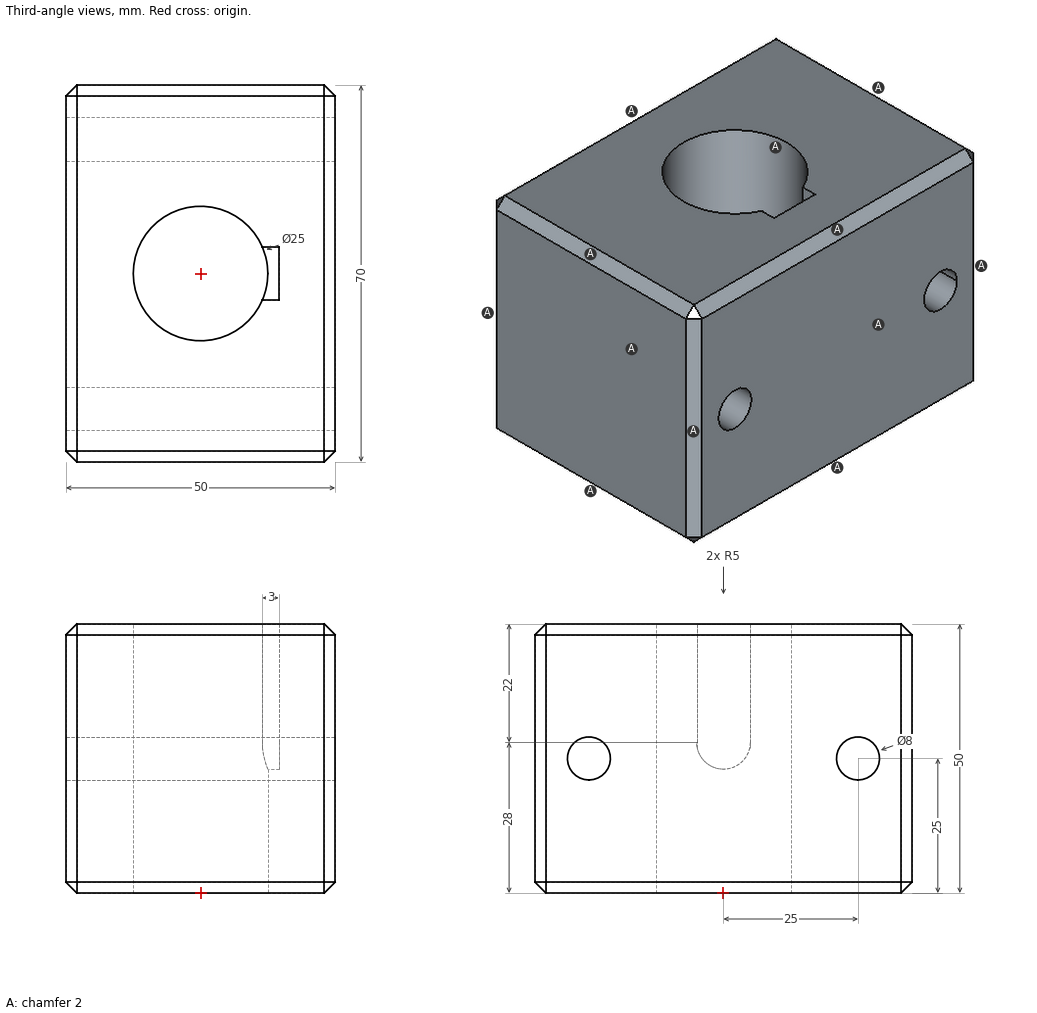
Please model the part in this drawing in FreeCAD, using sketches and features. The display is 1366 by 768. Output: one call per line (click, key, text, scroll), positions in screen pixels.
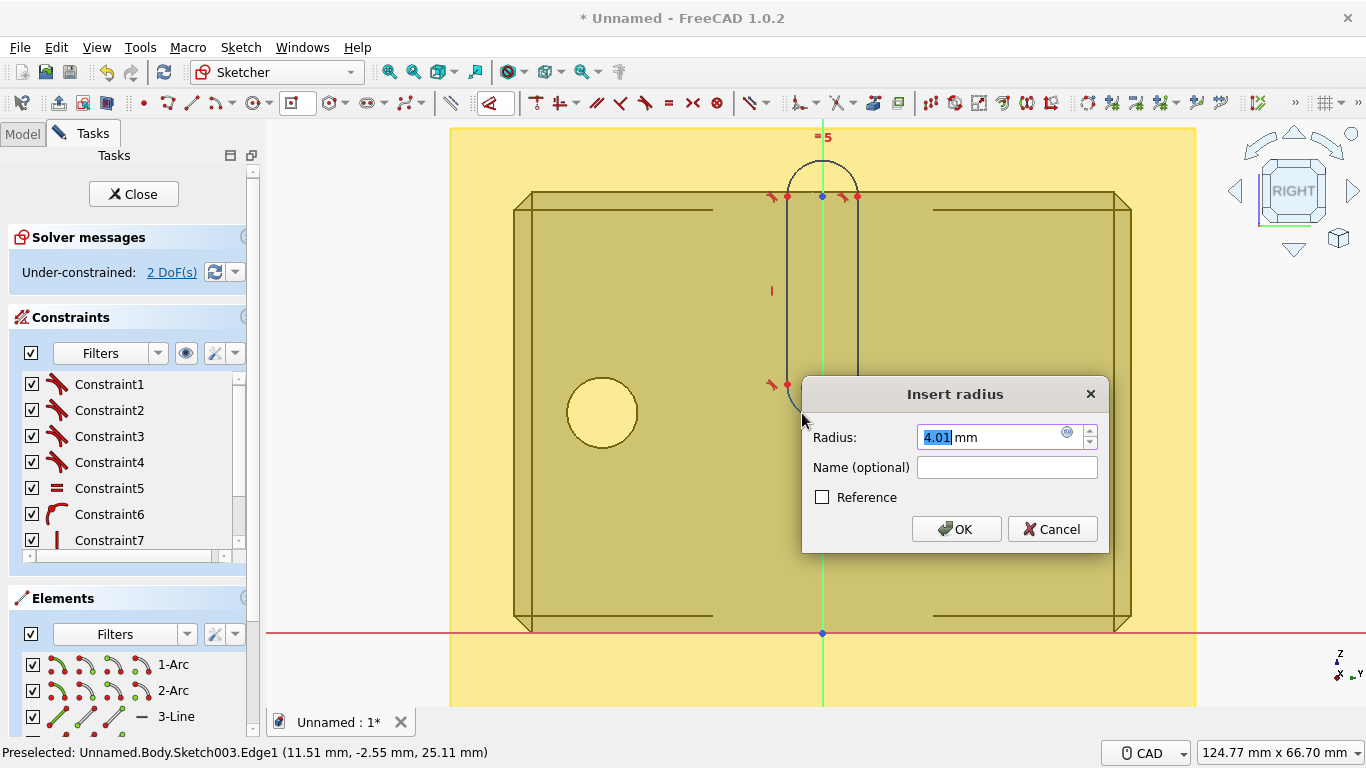
text(5)
key(Return)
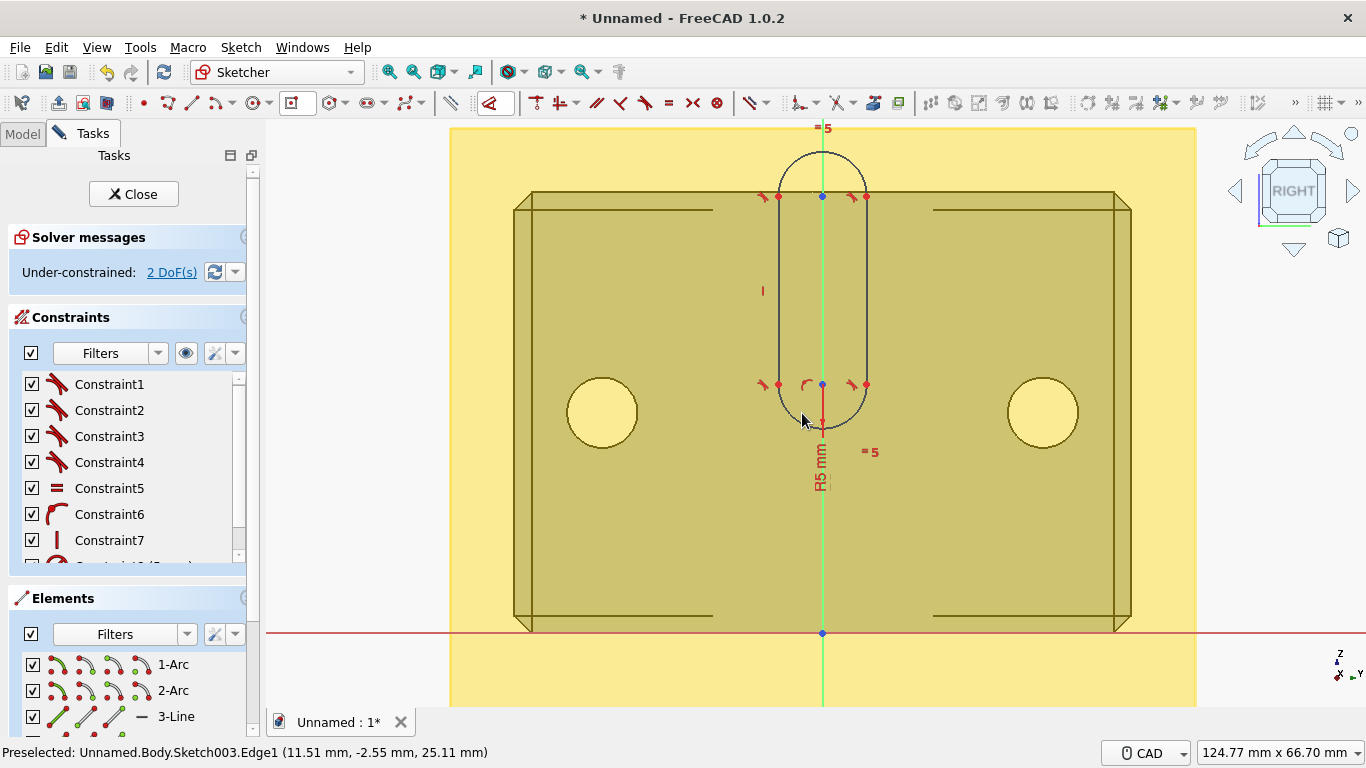
click(779, 328)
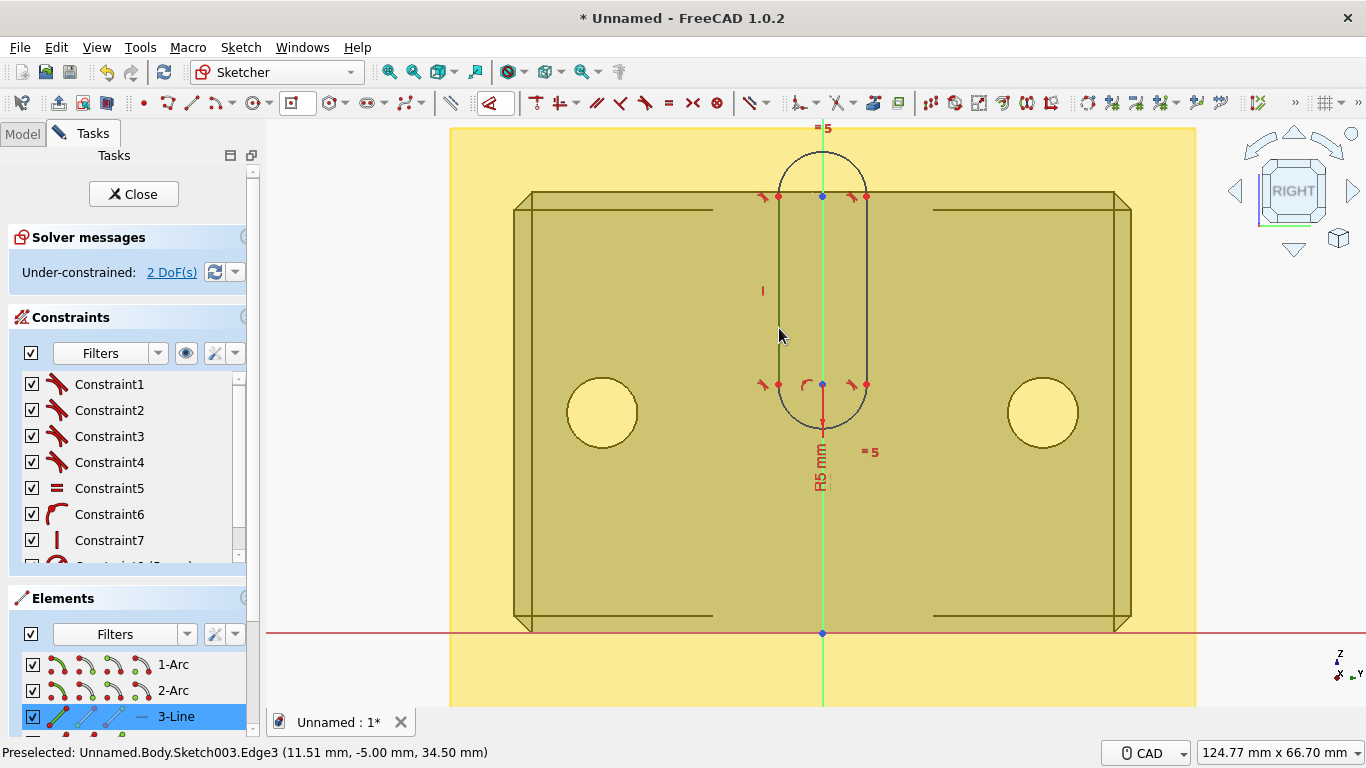
key(i)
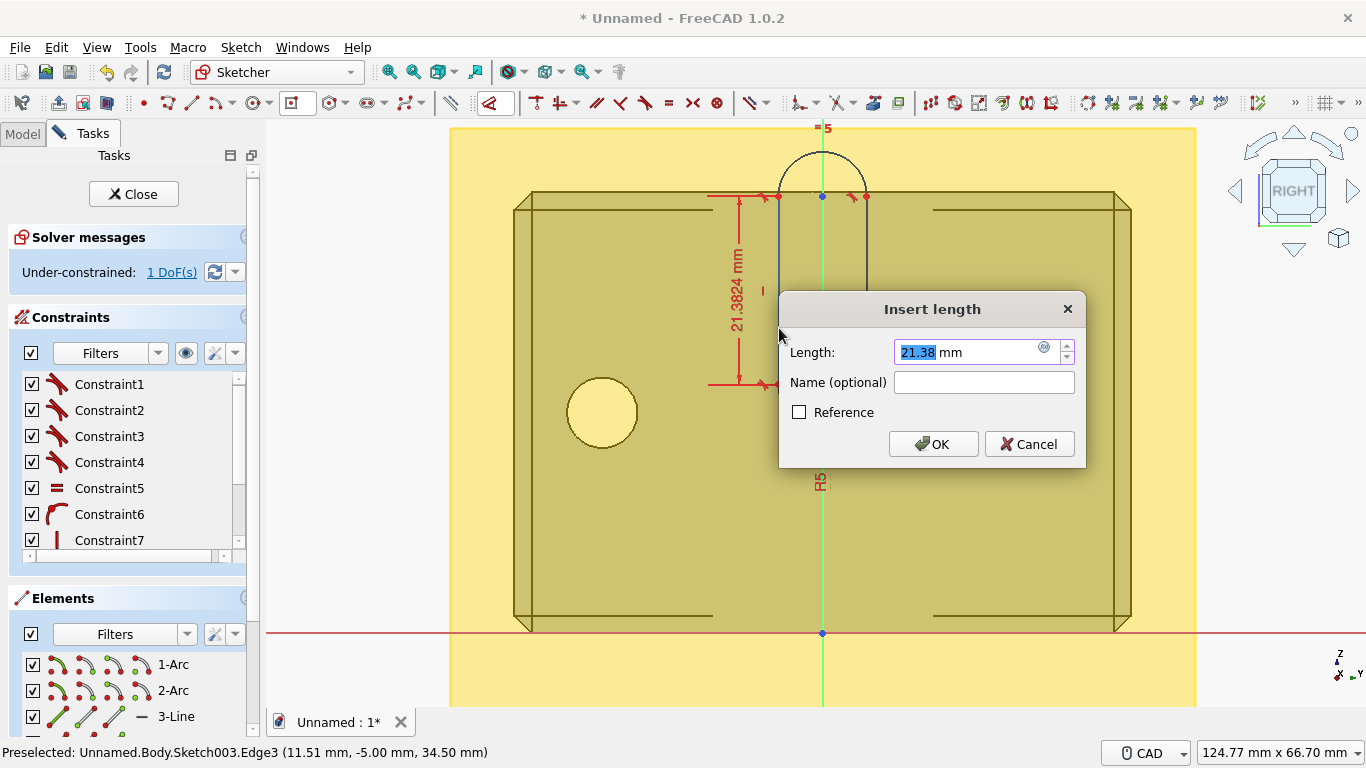
text(22)
key(Return)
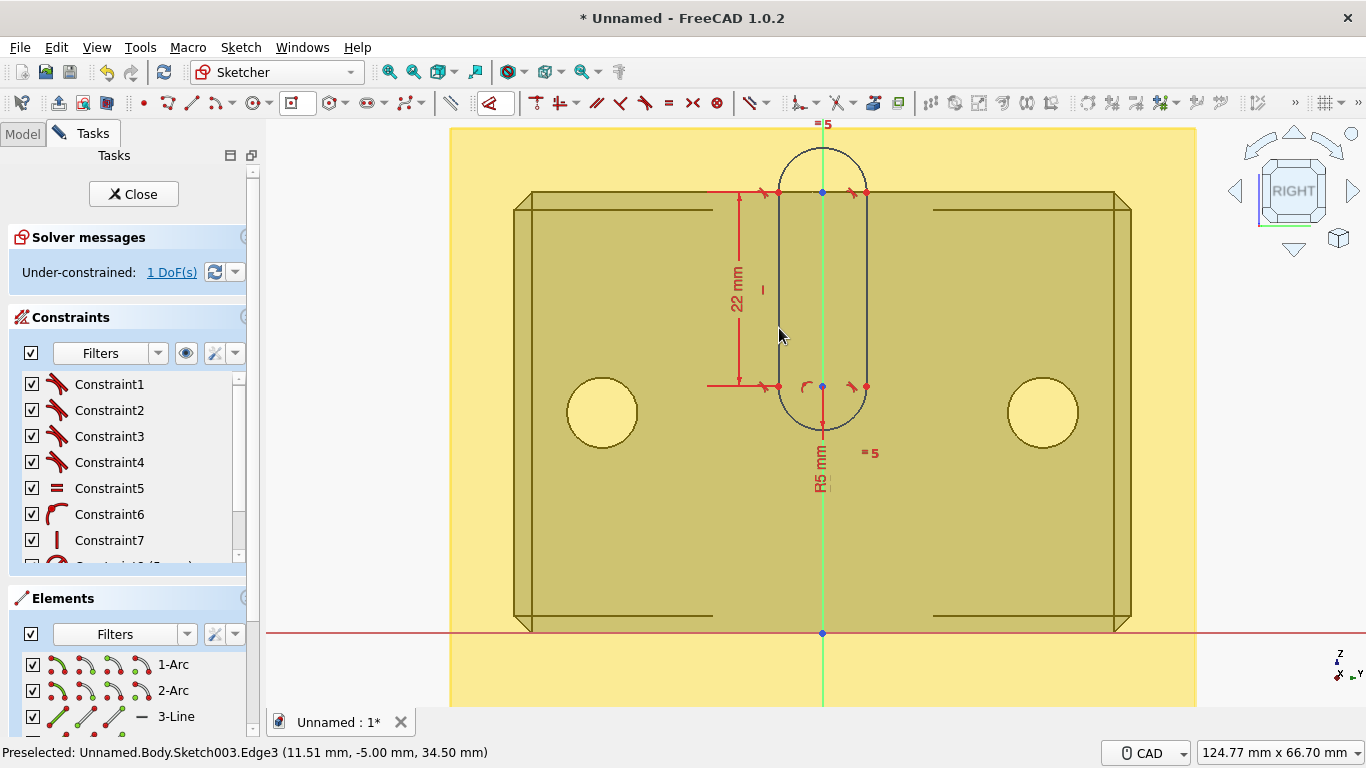
click(779, 386)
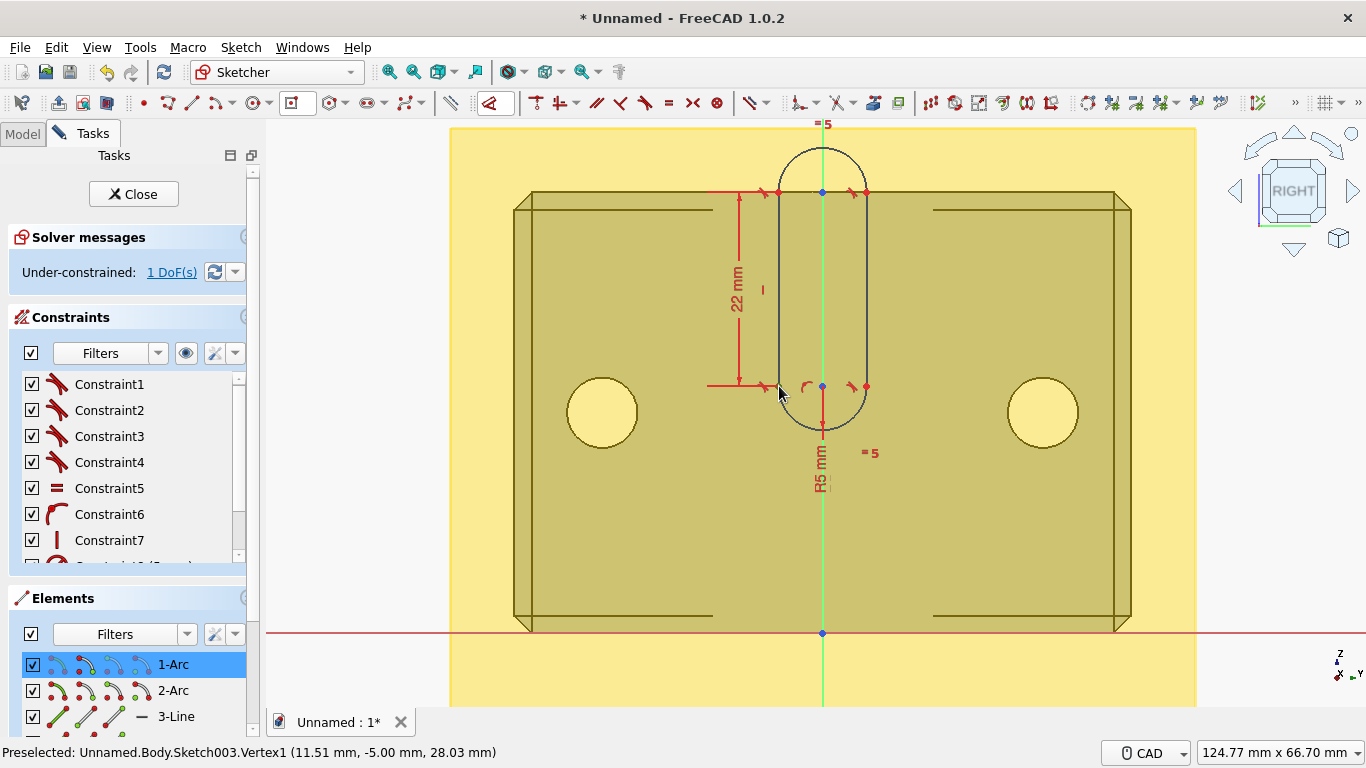
click(508, 104)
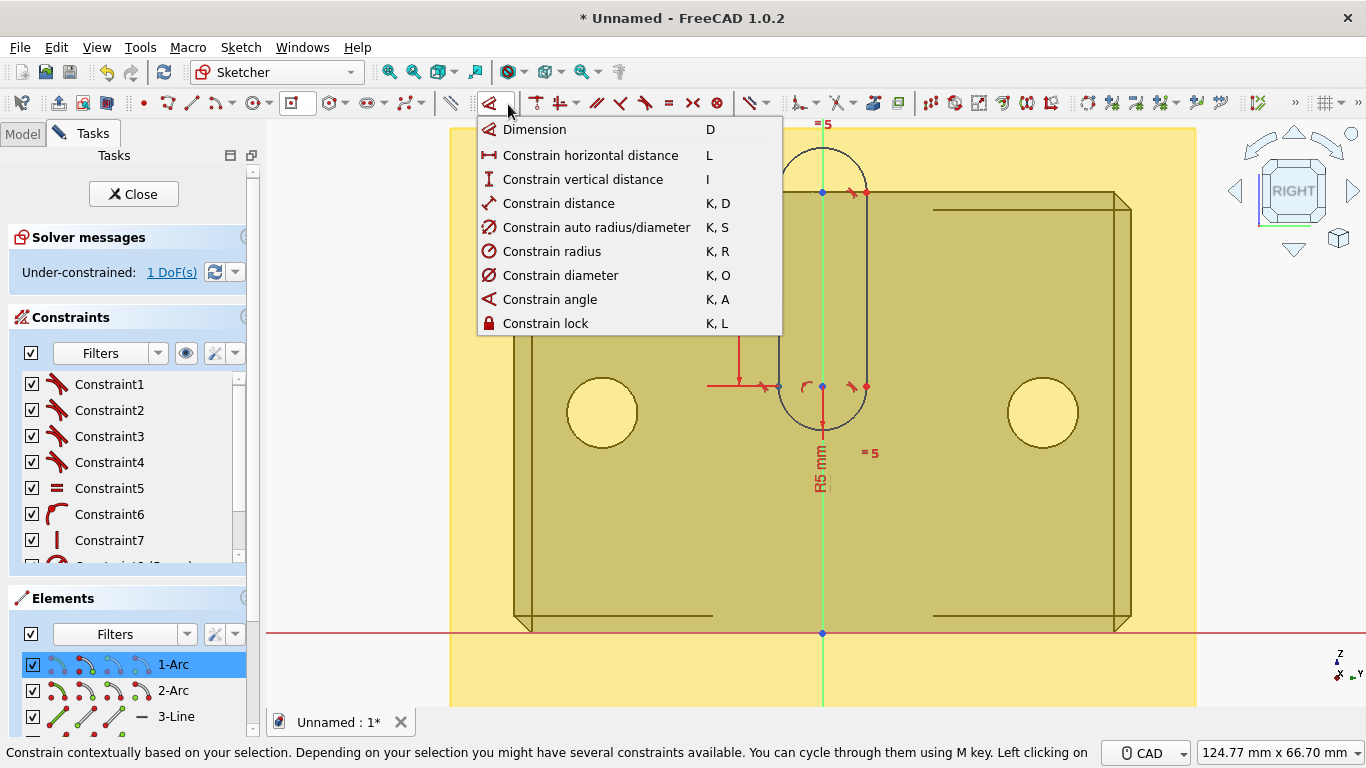
click(630, 179)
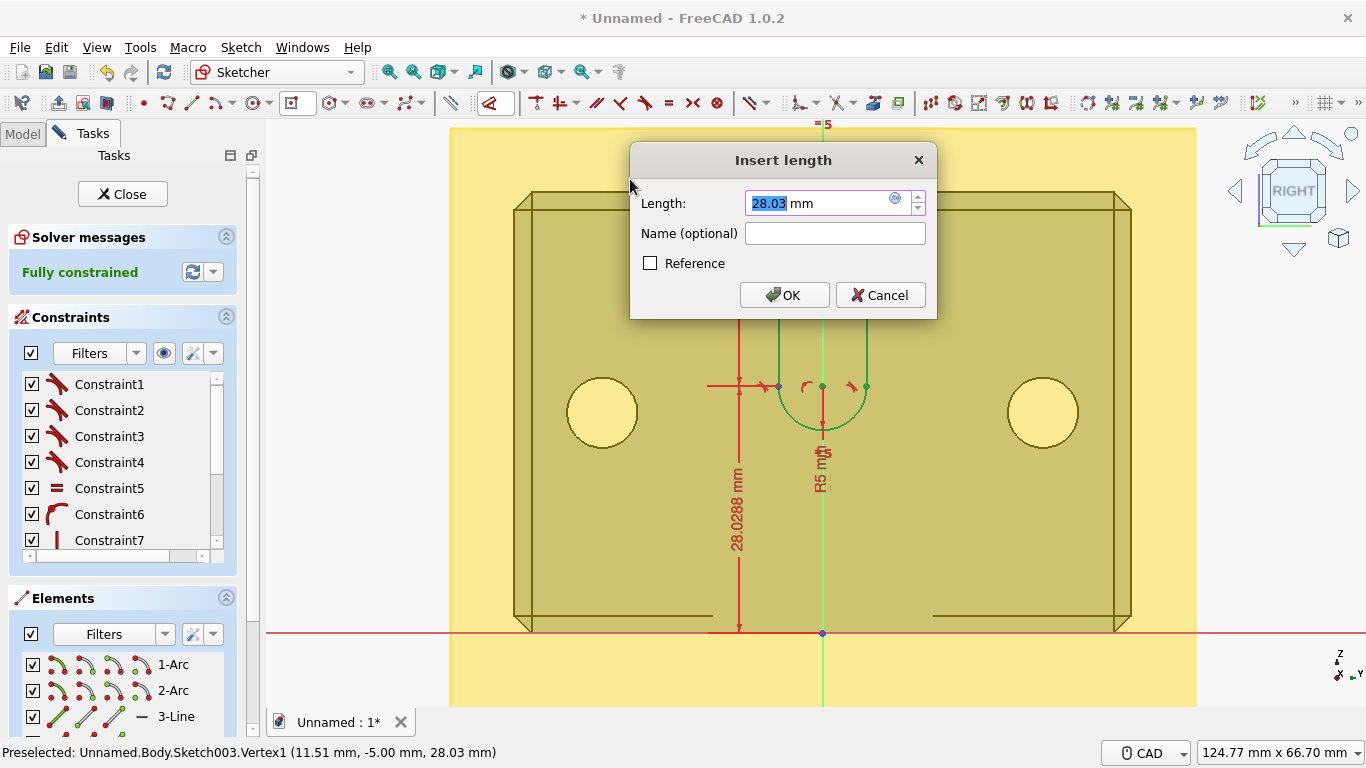
text(28)
key(Return)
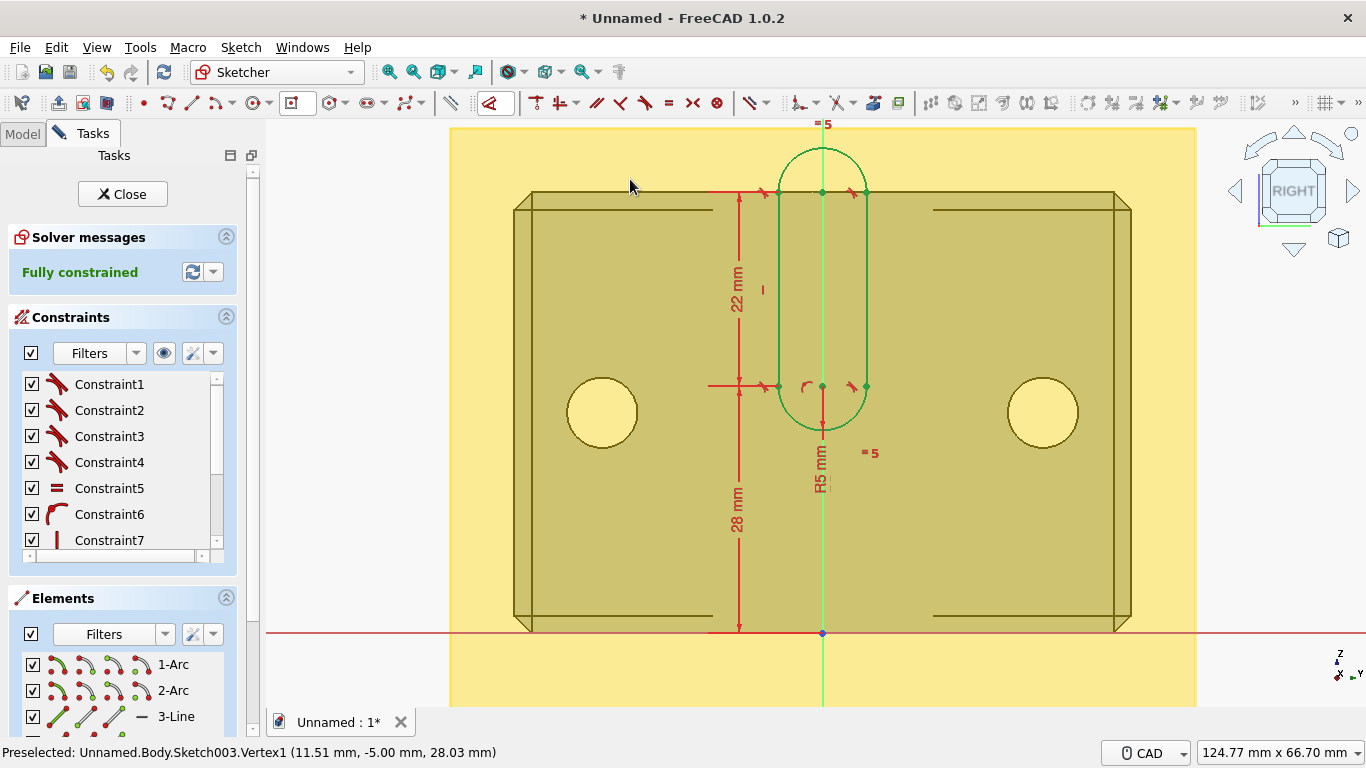
click(123, 194)